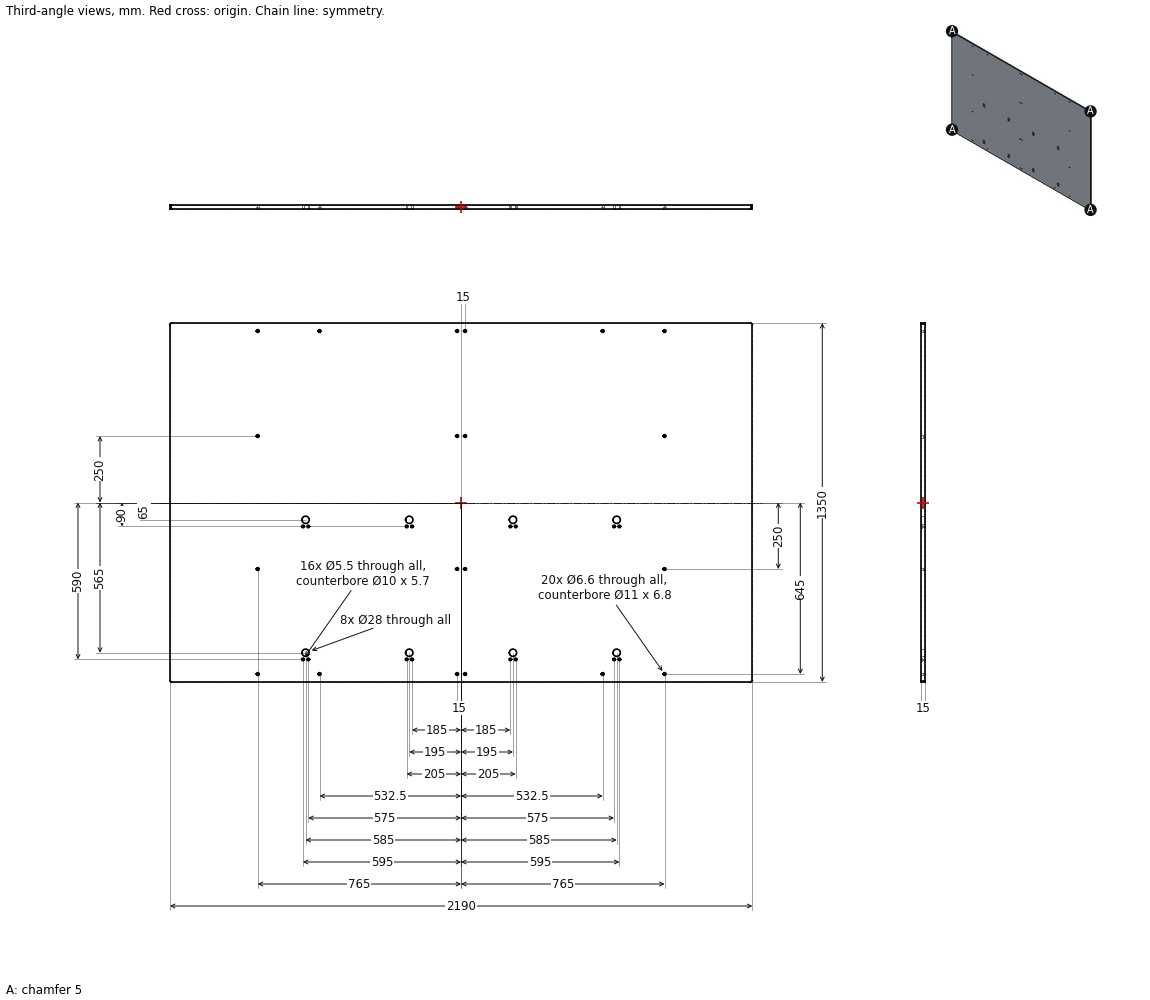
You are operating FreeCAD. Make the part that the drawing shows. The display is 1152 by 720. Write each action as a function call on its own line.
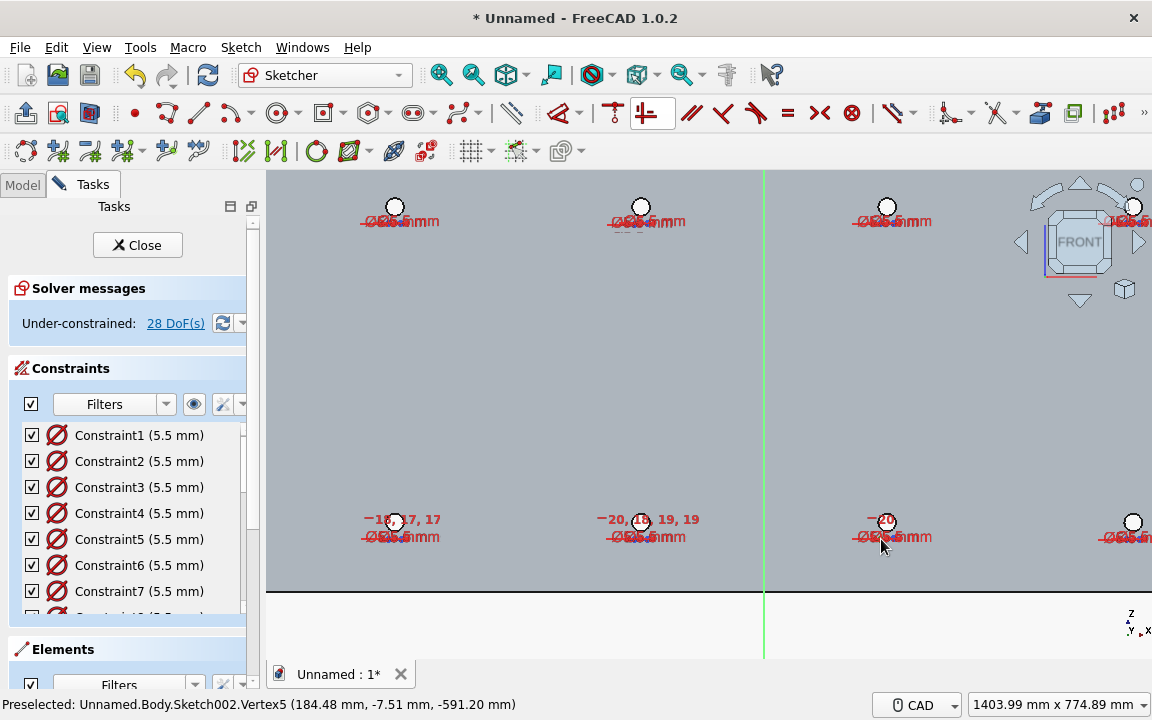
click(894, 539)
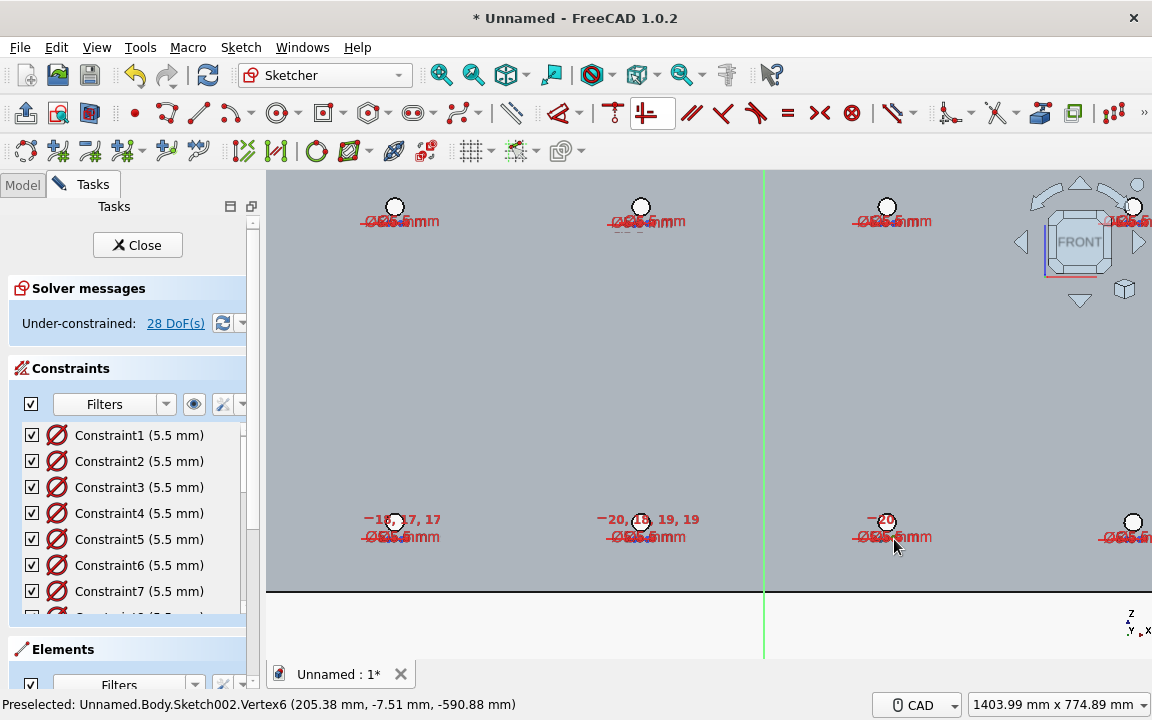
key(h)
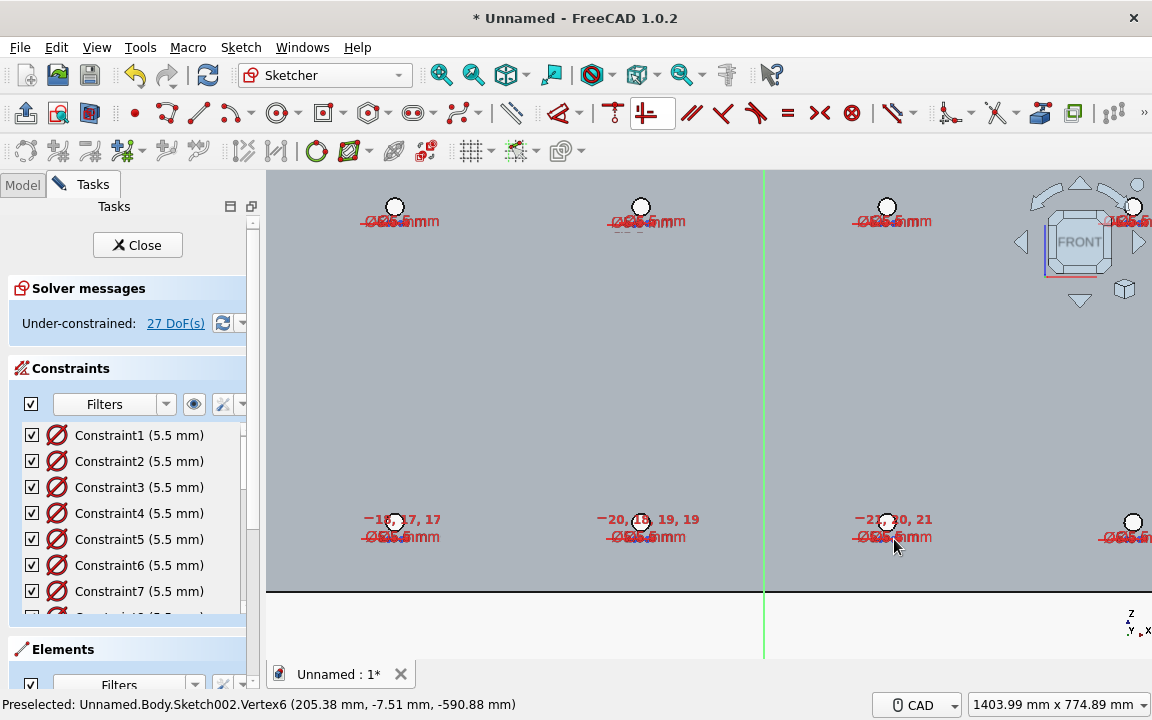
click(894, 539)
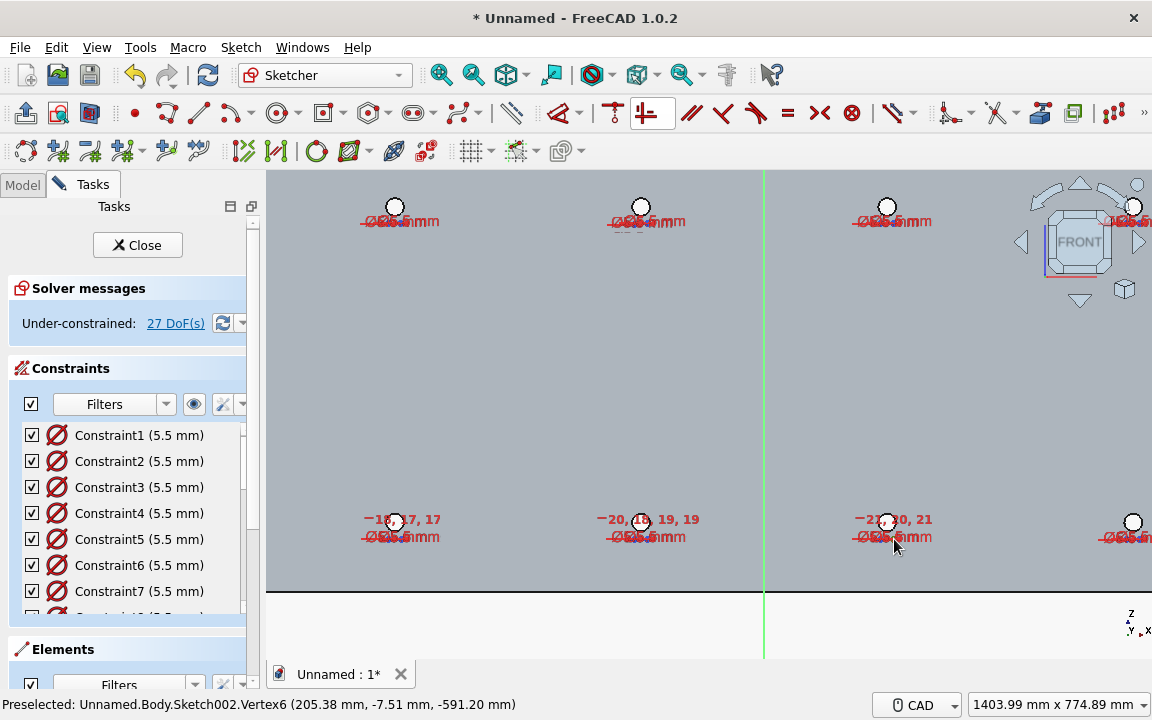
scroll(389, 540, down, 2)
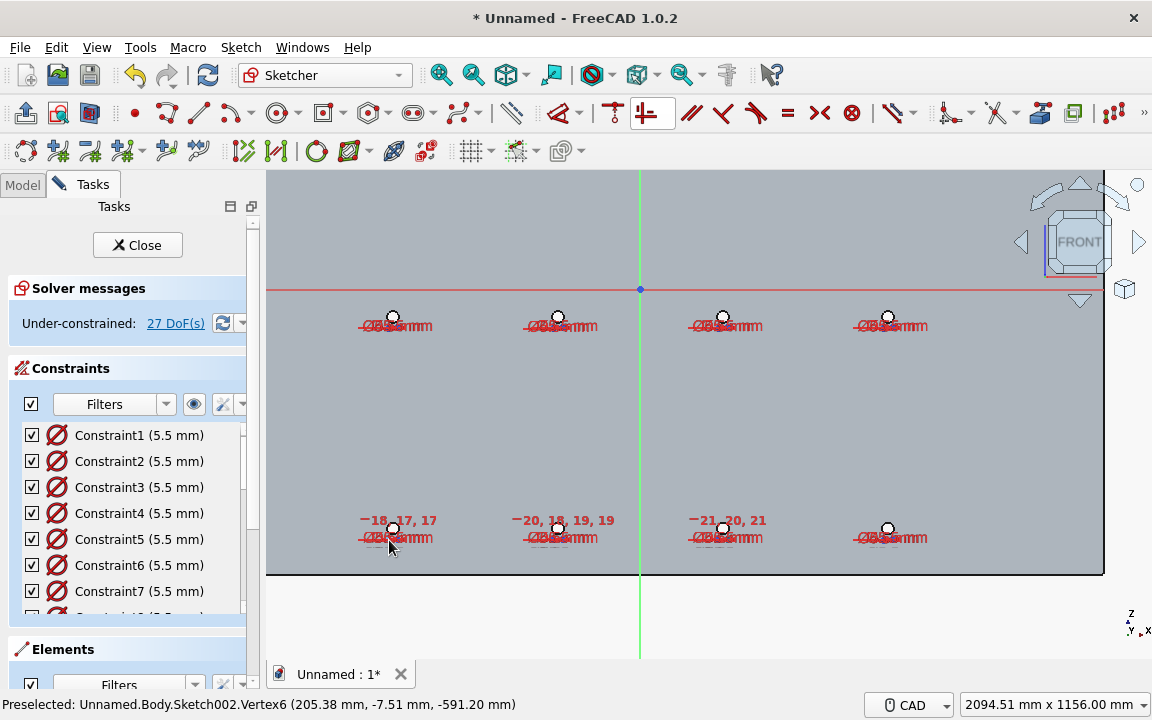
scroll(884, 540, up, 2)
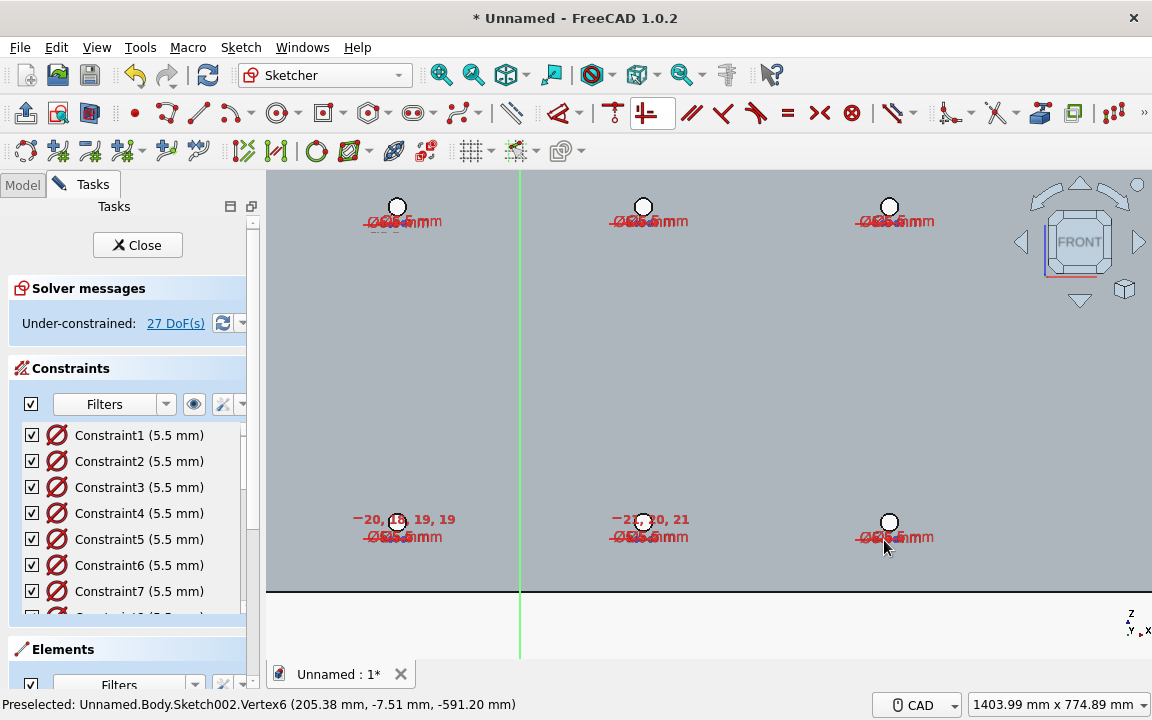
click(883, 540)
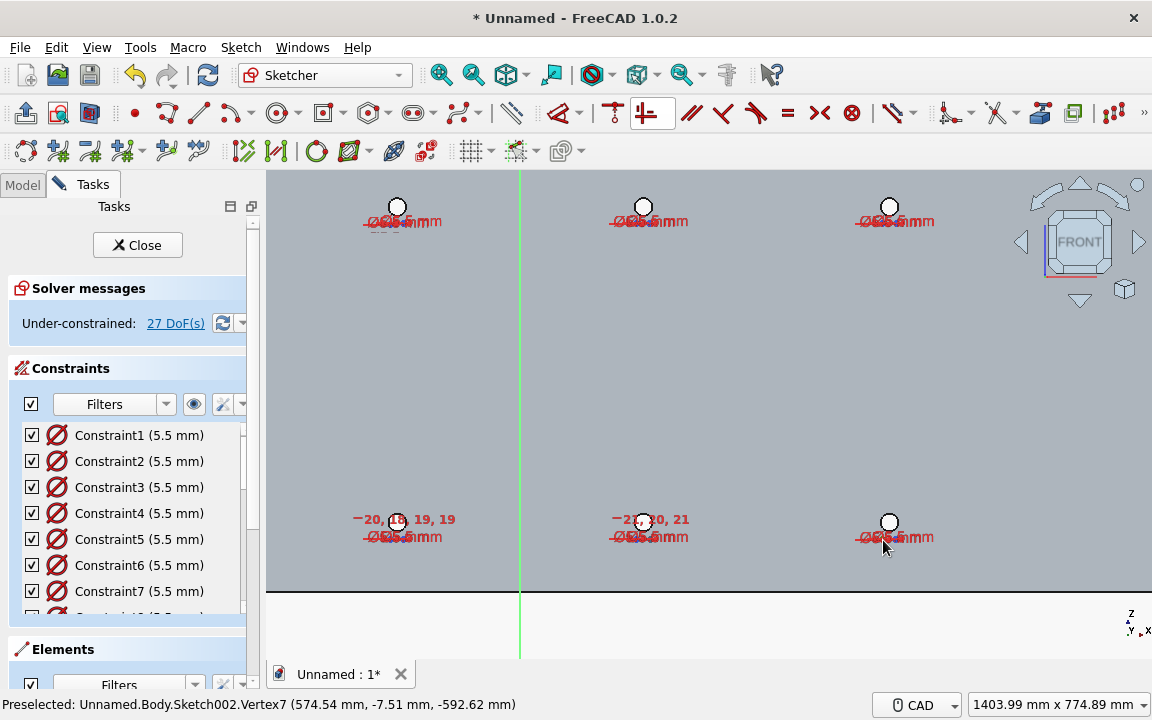
key(h)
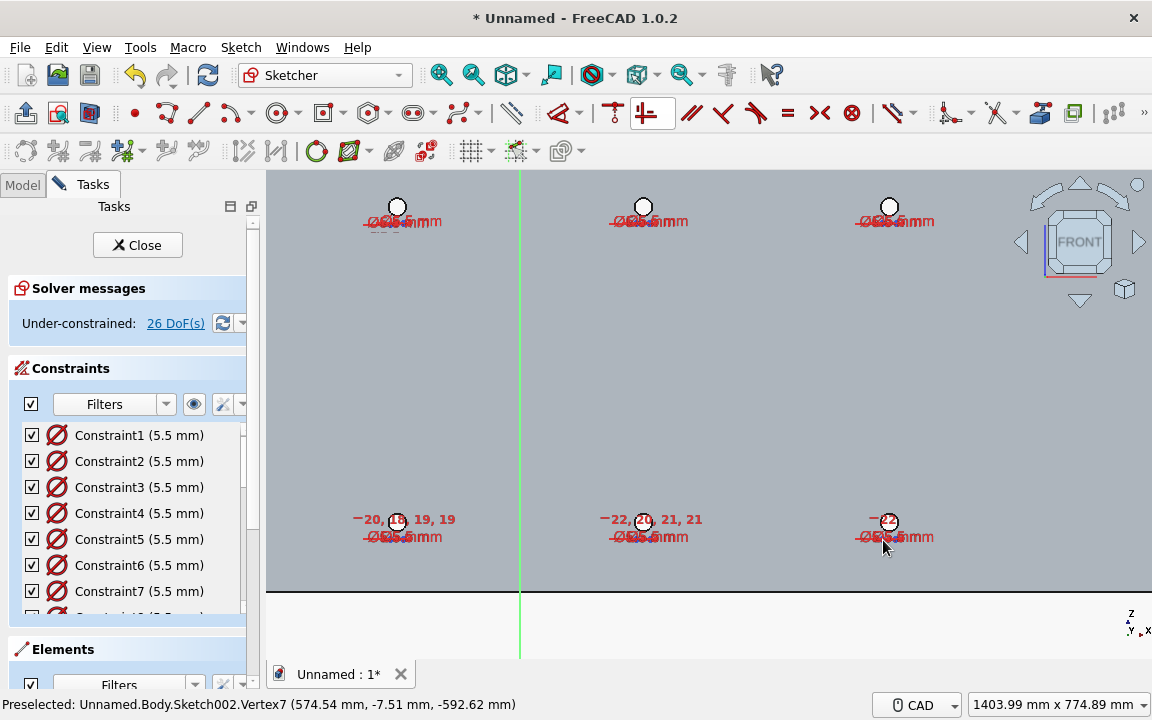
click(883, 539)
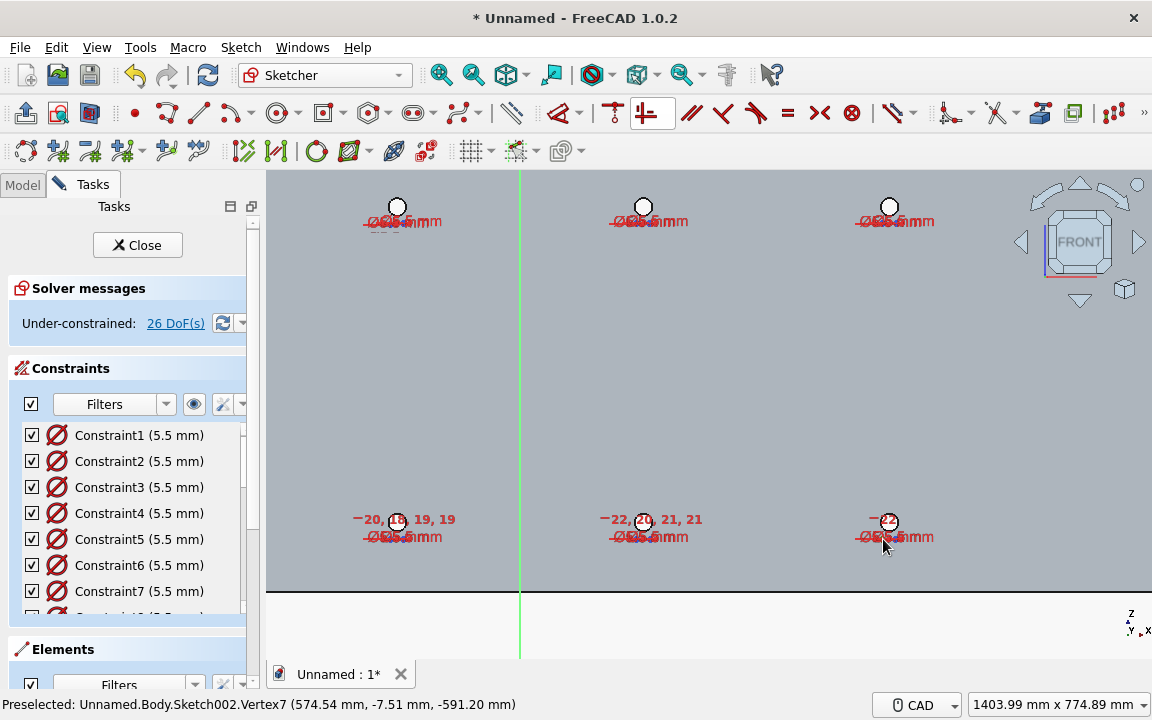
click(896, 539)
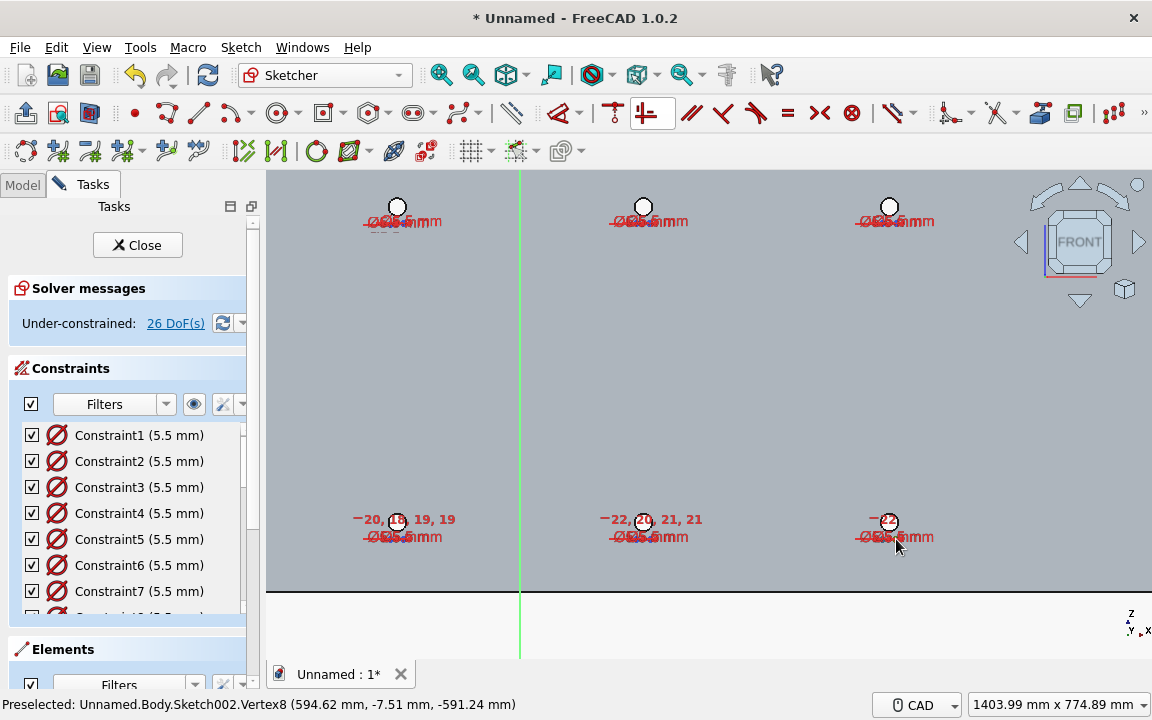
key(h)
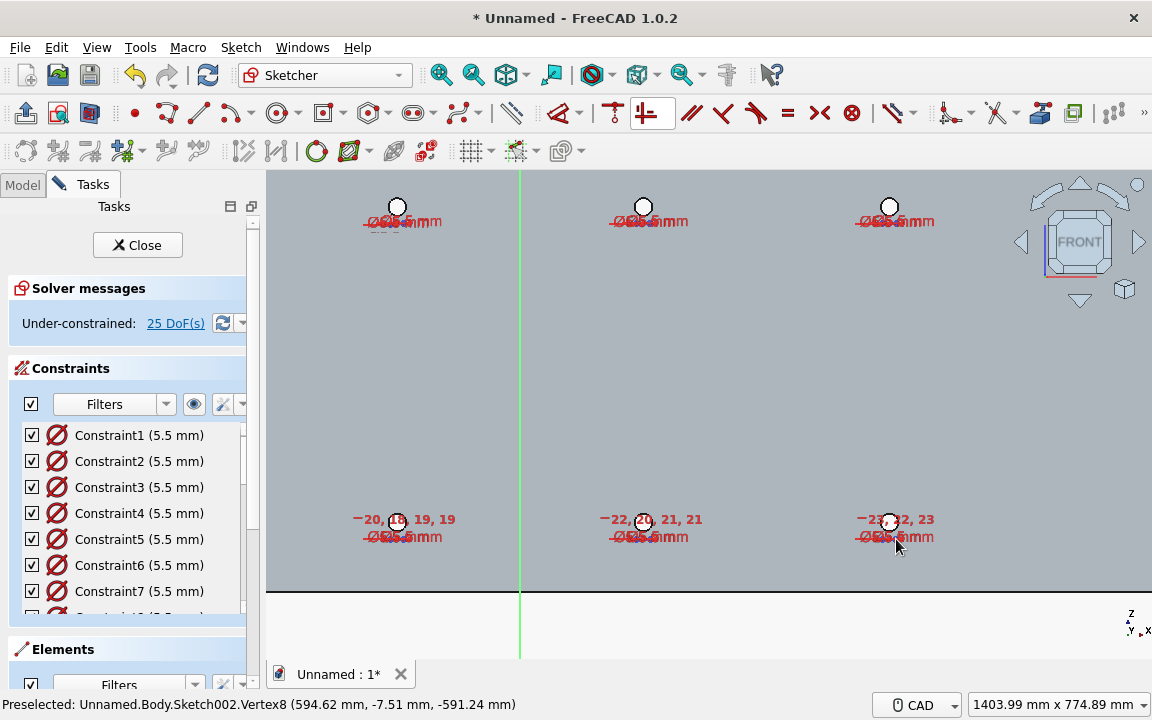
click(391, 539)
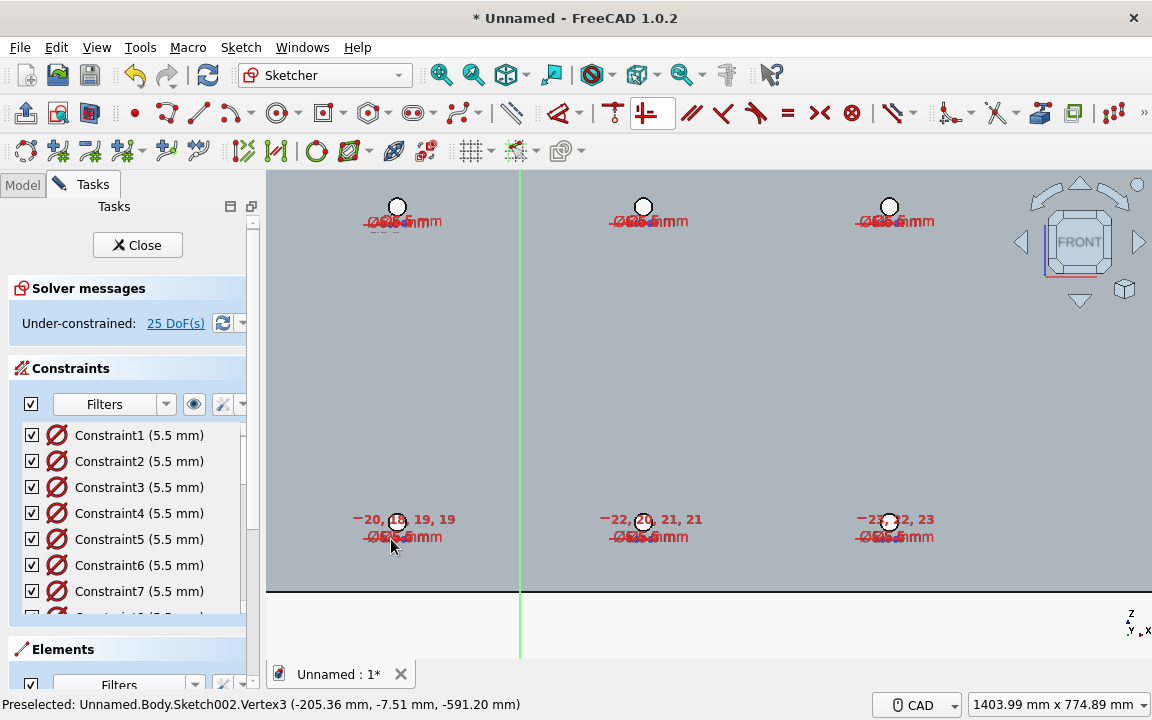
click(391, 225)